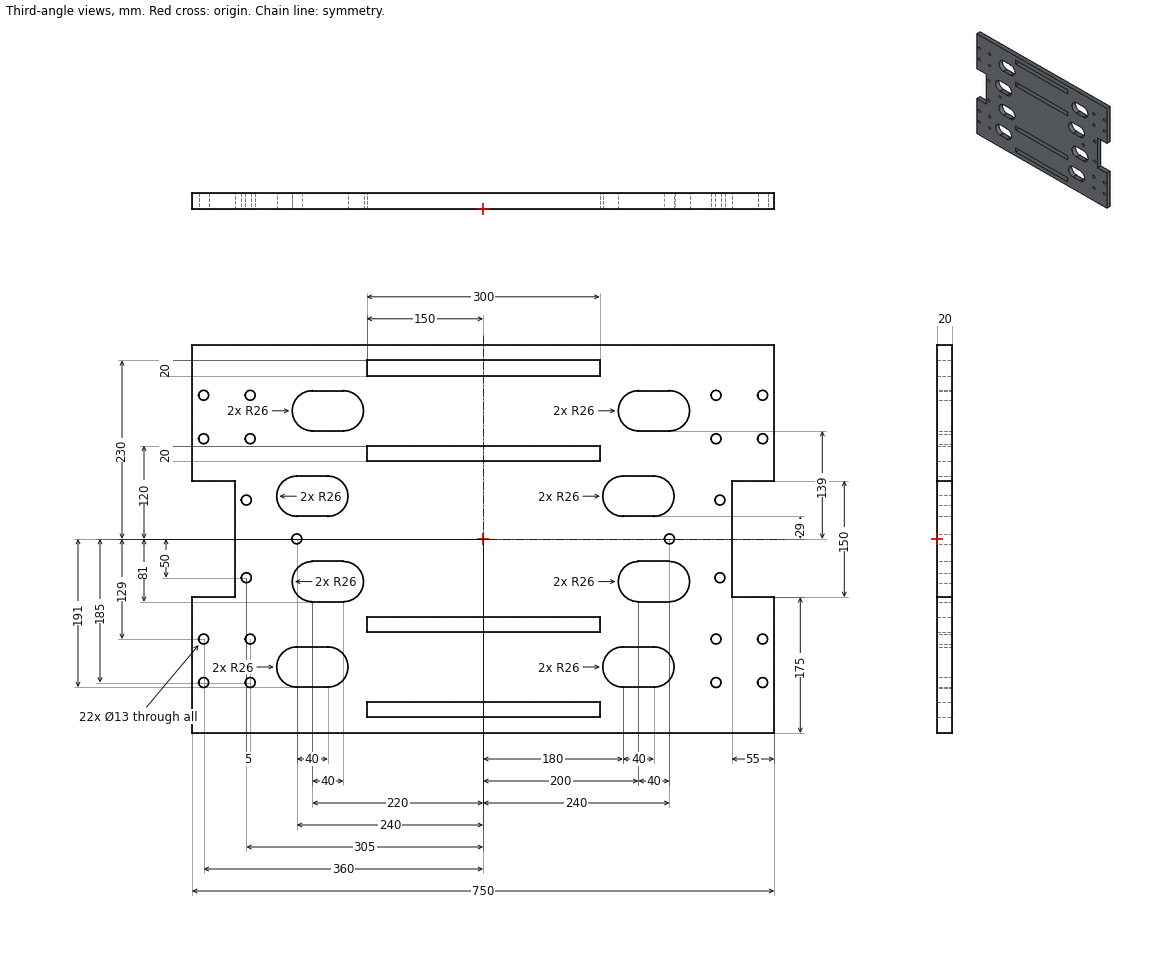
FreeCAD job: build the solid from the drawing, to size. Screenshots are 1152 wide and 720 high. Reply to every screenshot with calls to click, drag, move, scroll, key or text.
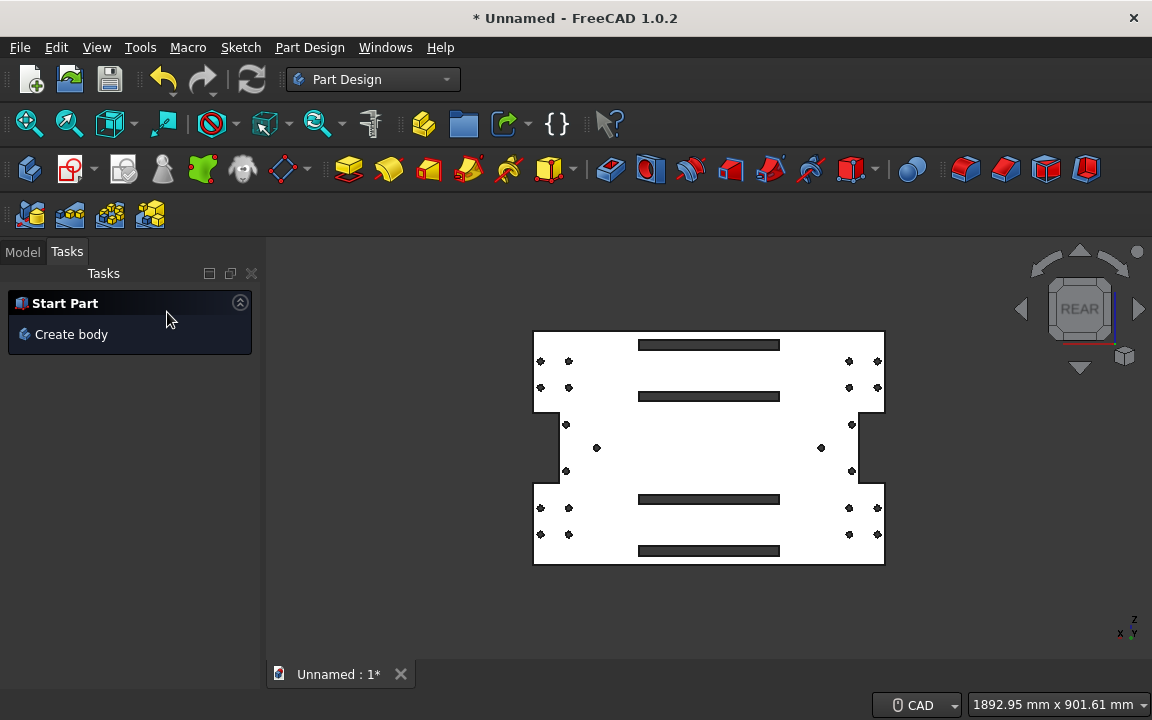
click(659, 447)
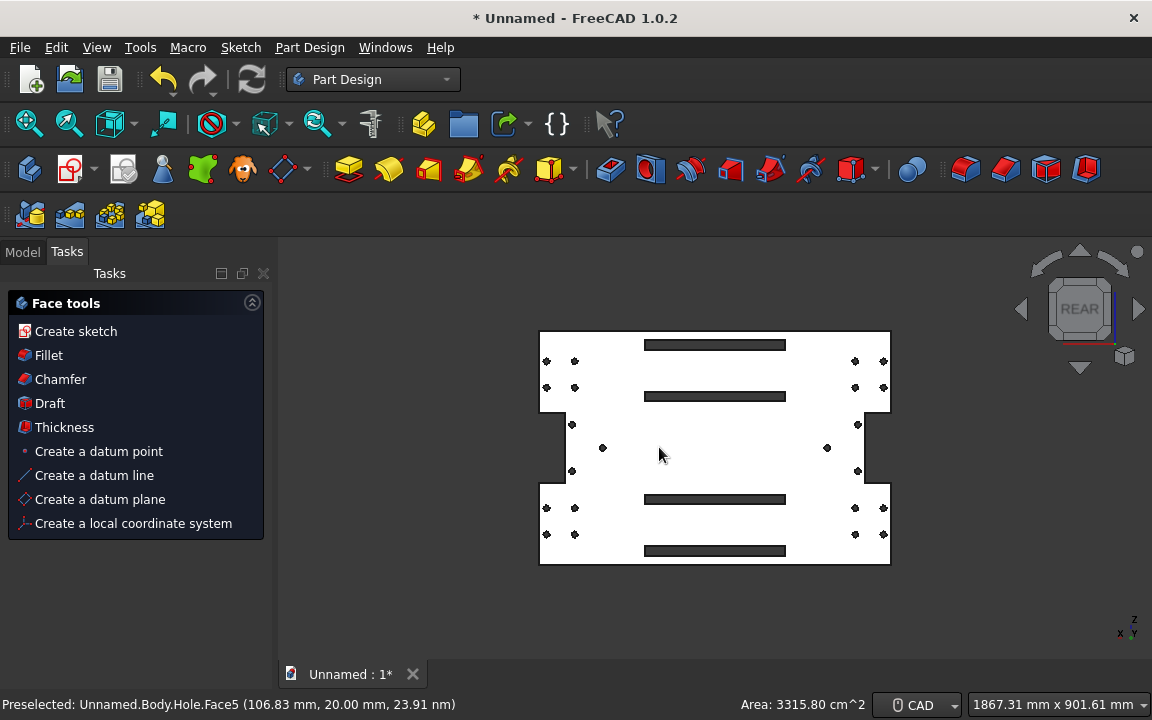
click(70, 170)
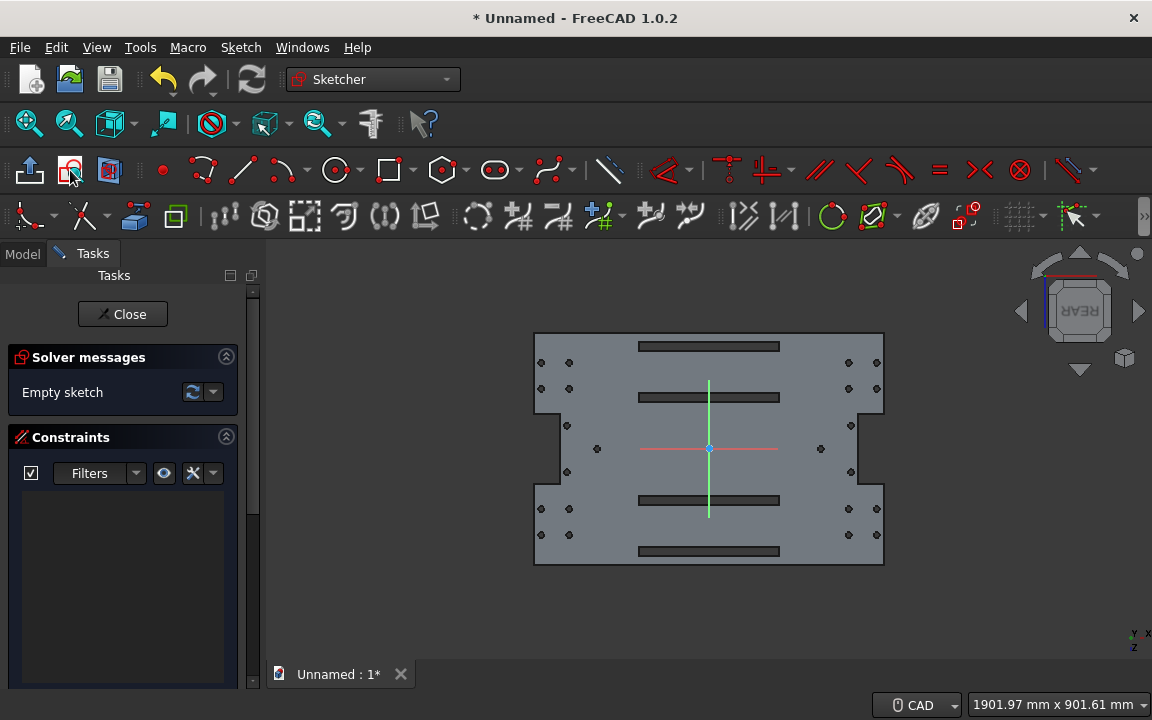
scroll(603, 364, up, 12)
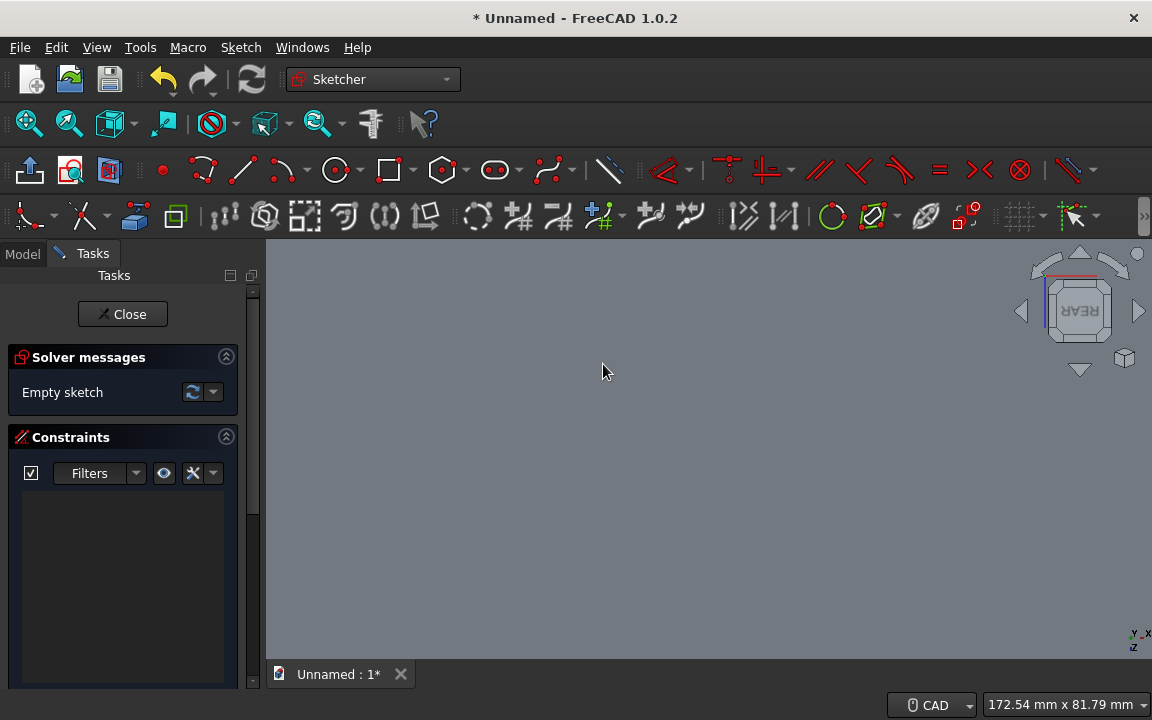
click(496, 170)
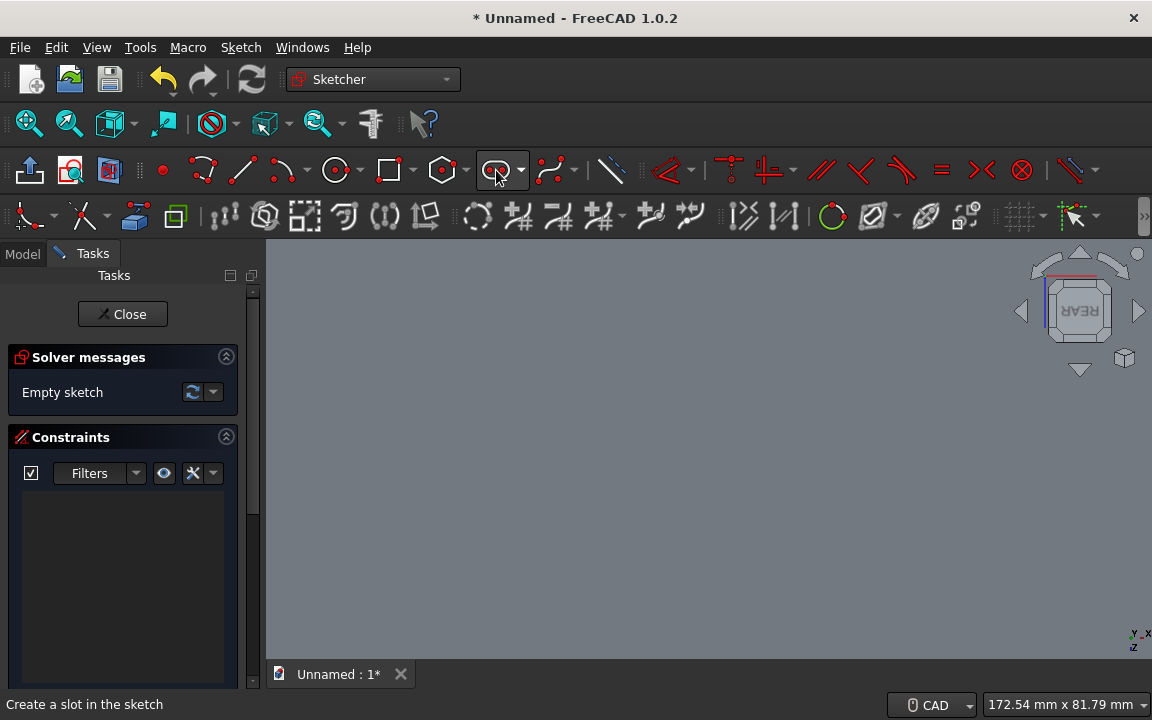
click(535, 451)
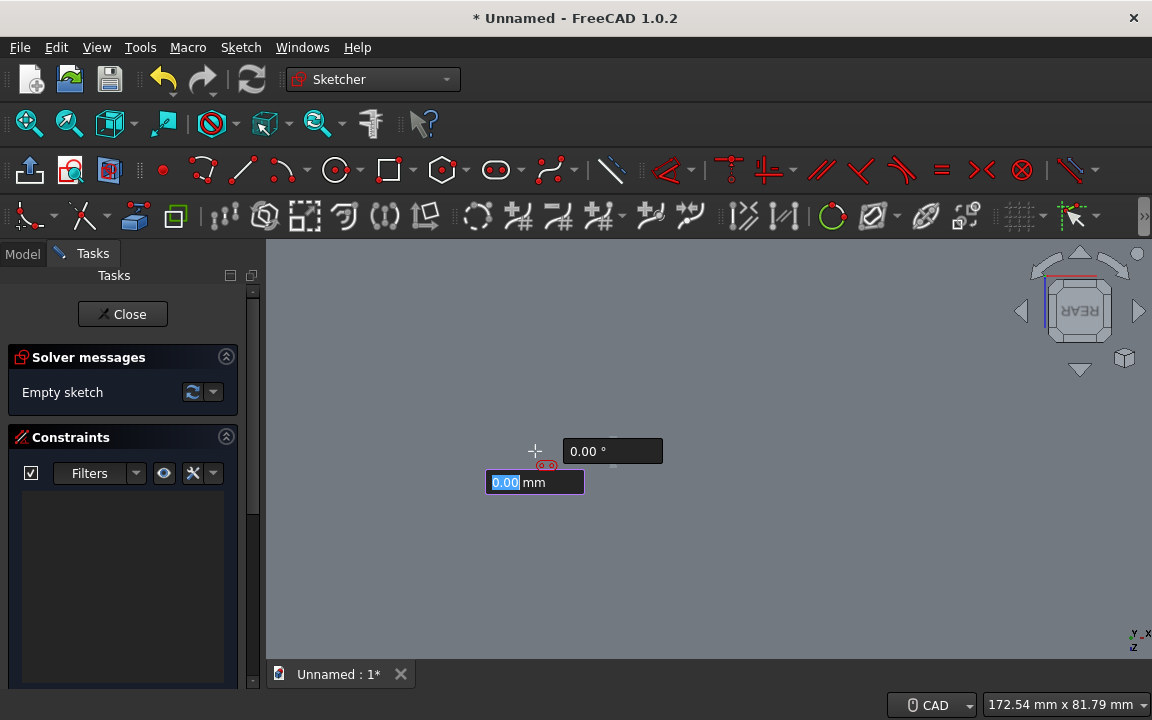
click(741, 451)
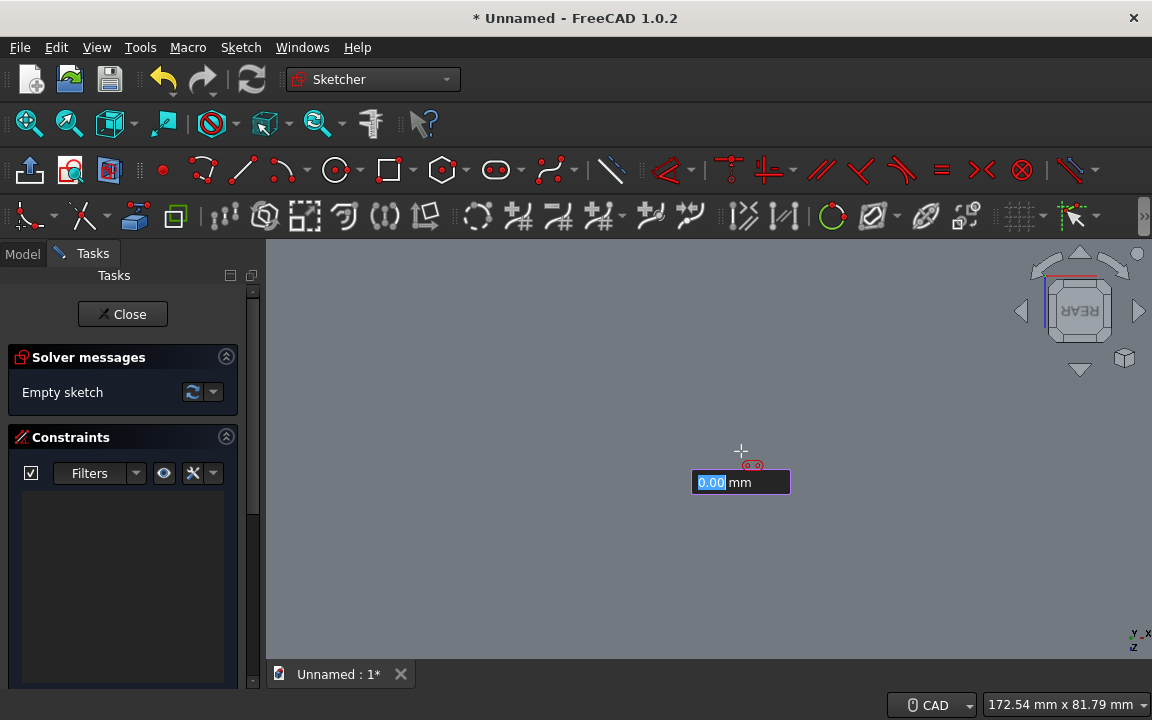
click(638, 317)
key(Escape)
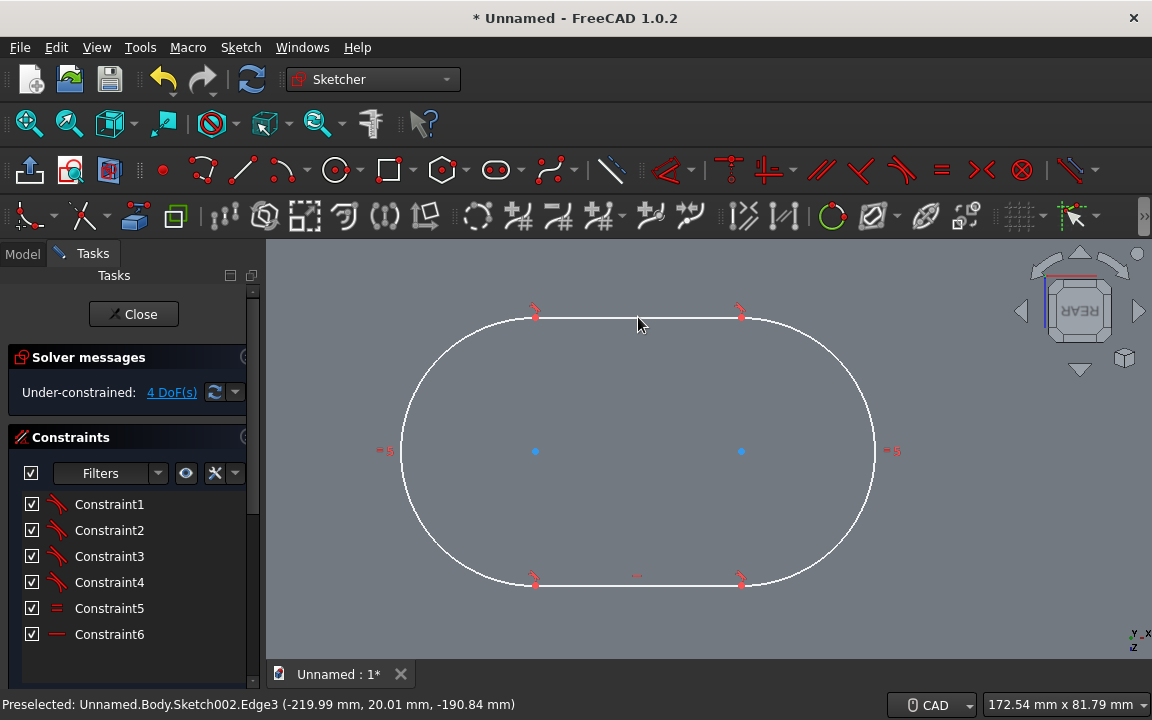
click(666, 170)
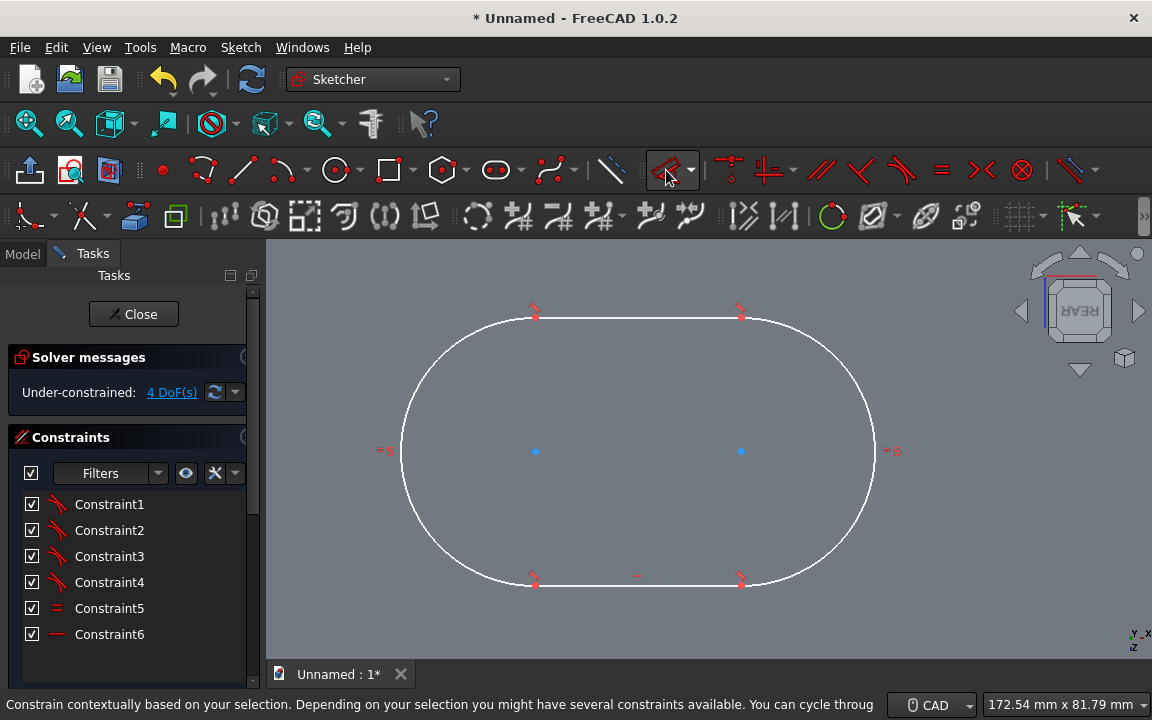
click(427, 373)
click(401, 354)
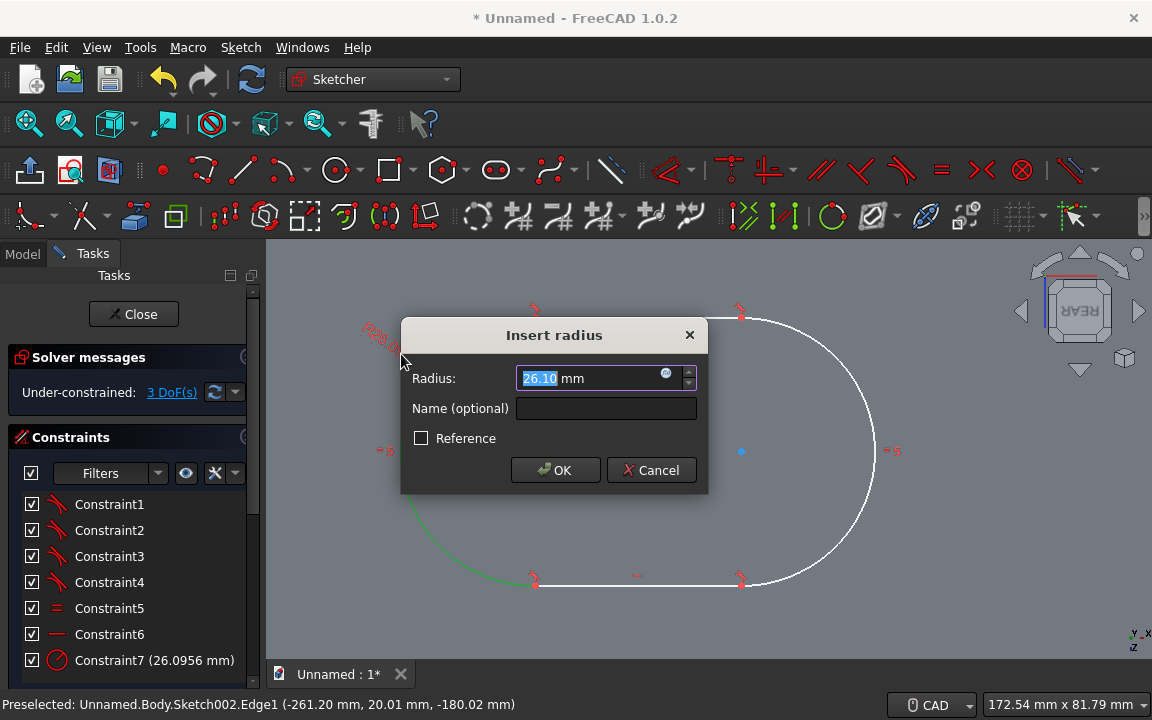
text(26)
key(Return)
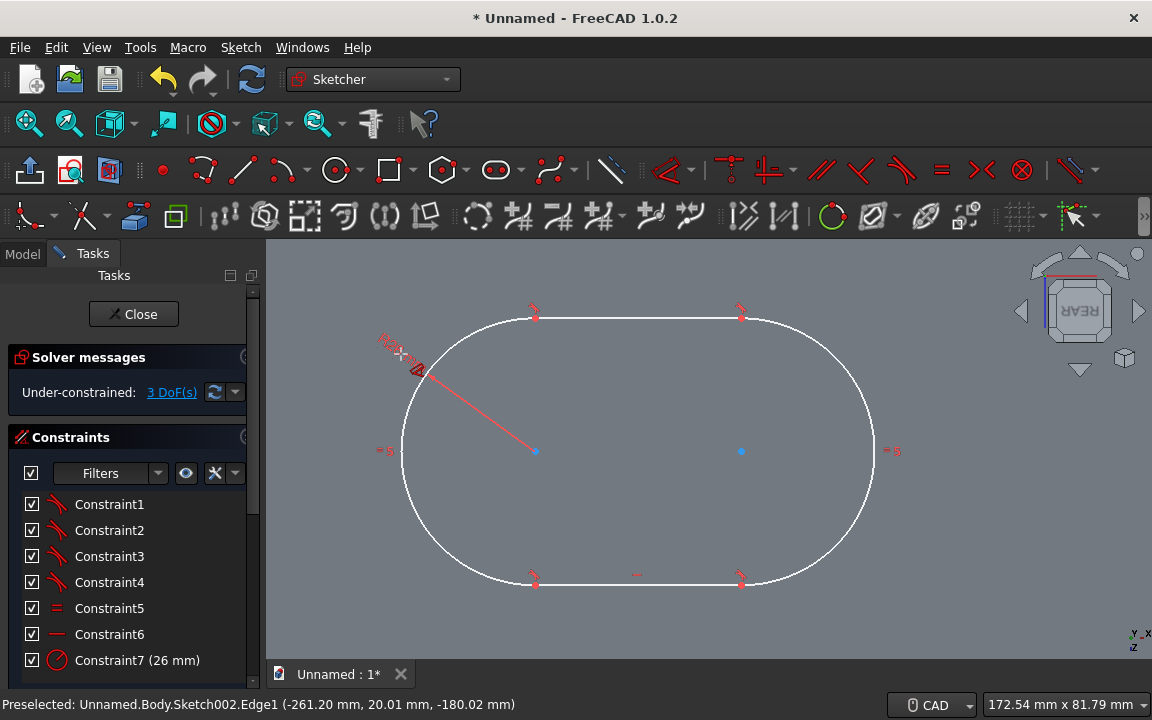
click(597, 318)
click(638, 284)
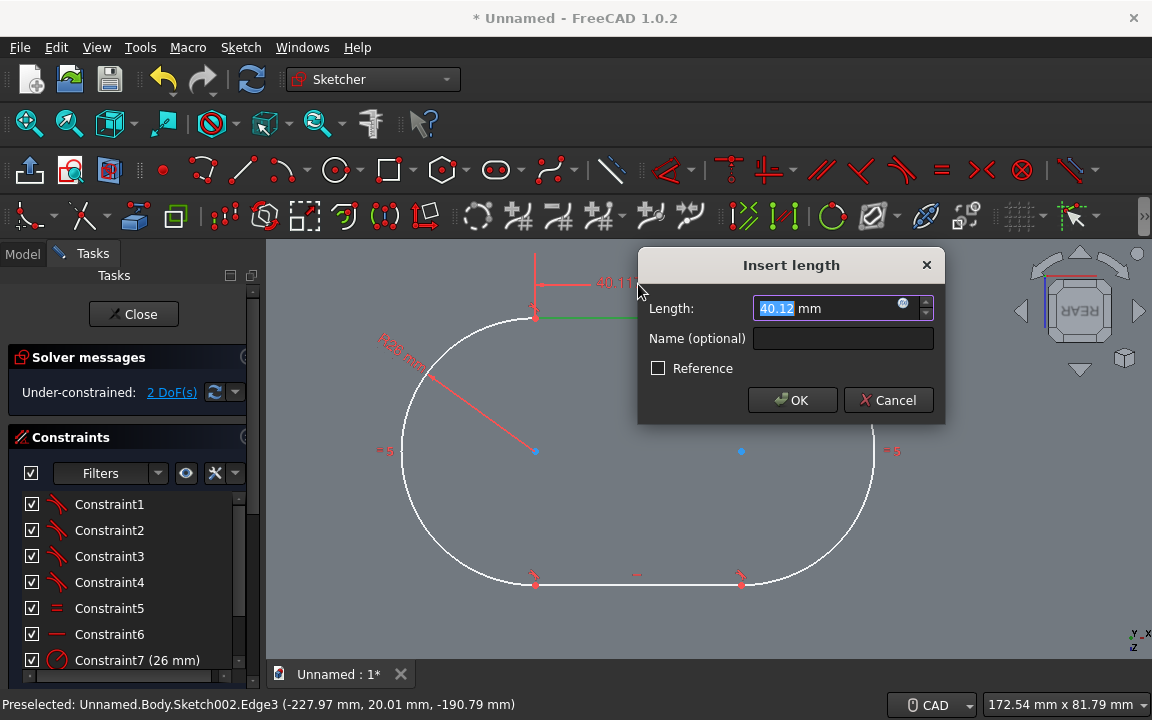
text(40)
key(Return)